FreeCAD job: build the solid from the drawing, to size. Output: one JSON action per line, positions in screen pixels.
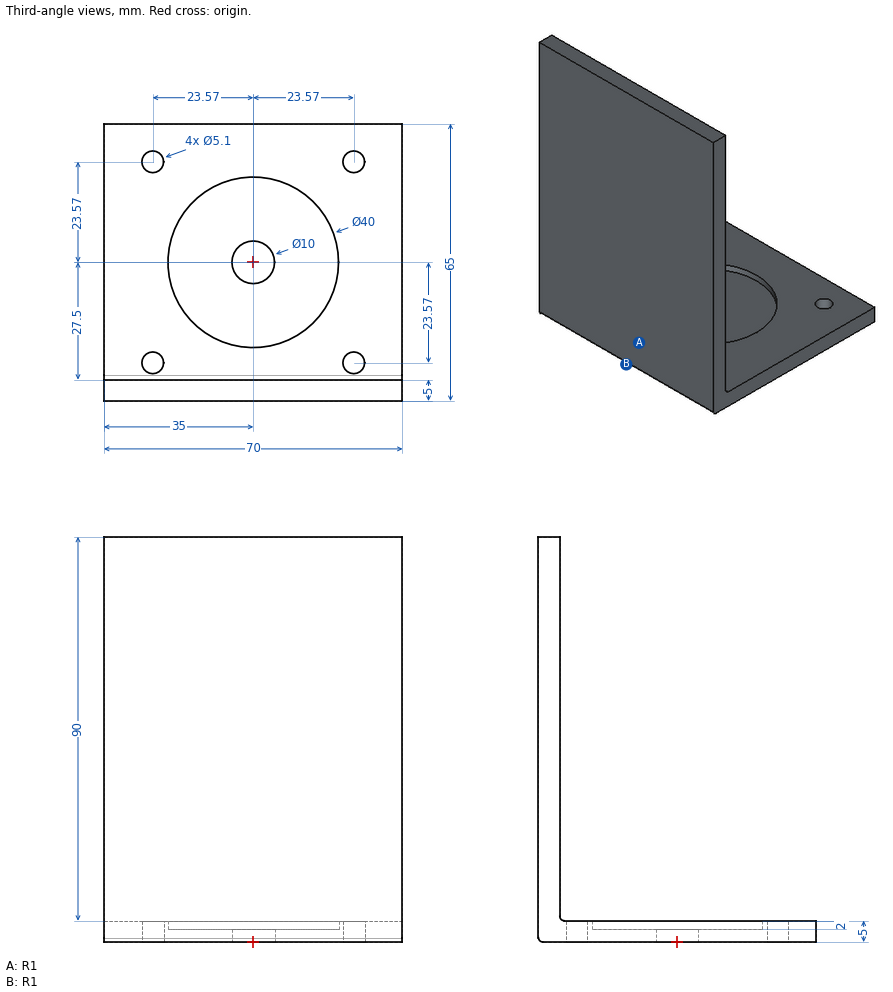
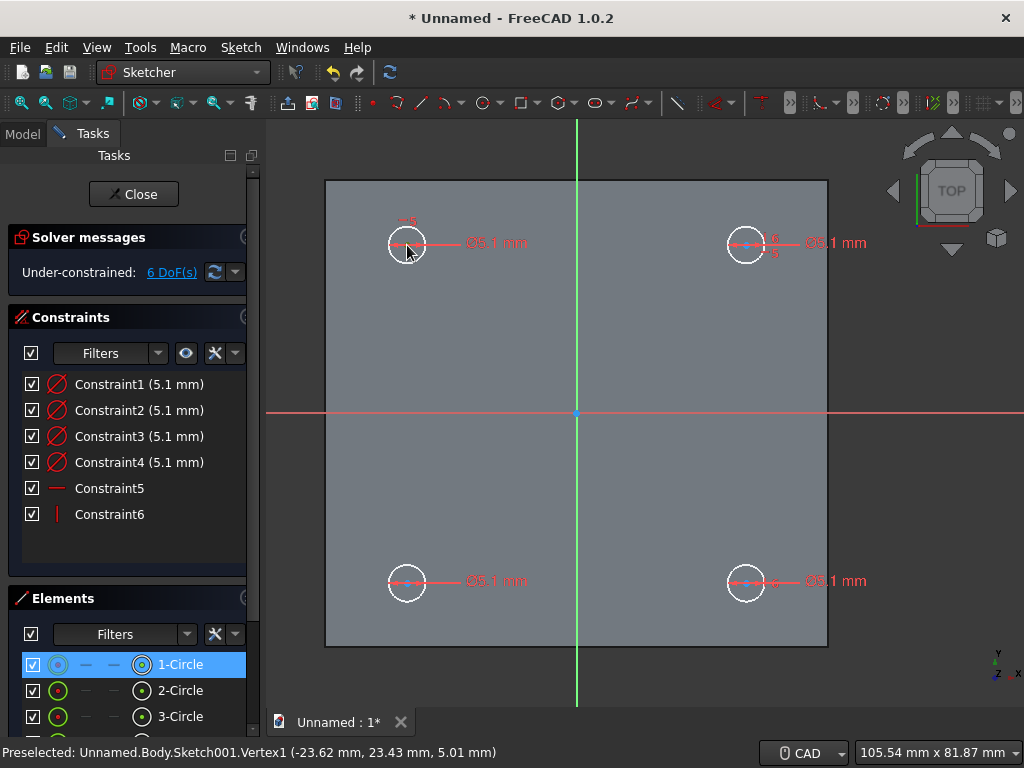
{"action": "left_click", "coordinate": [407, 583]}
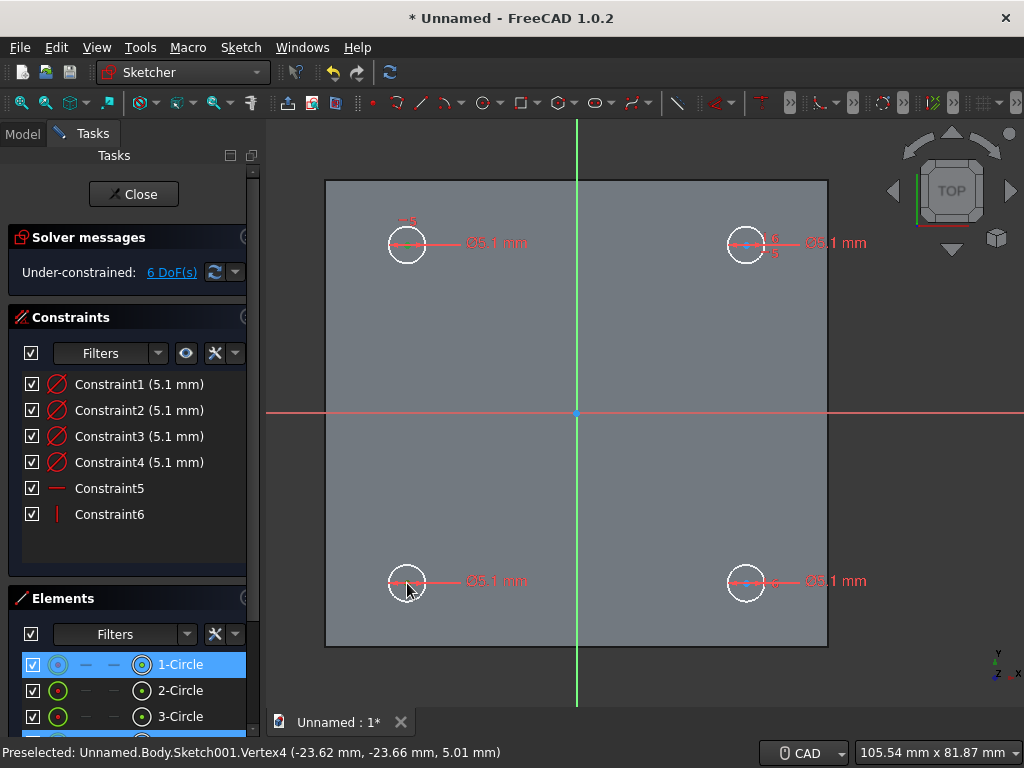
{"action": "key", "text": "v"}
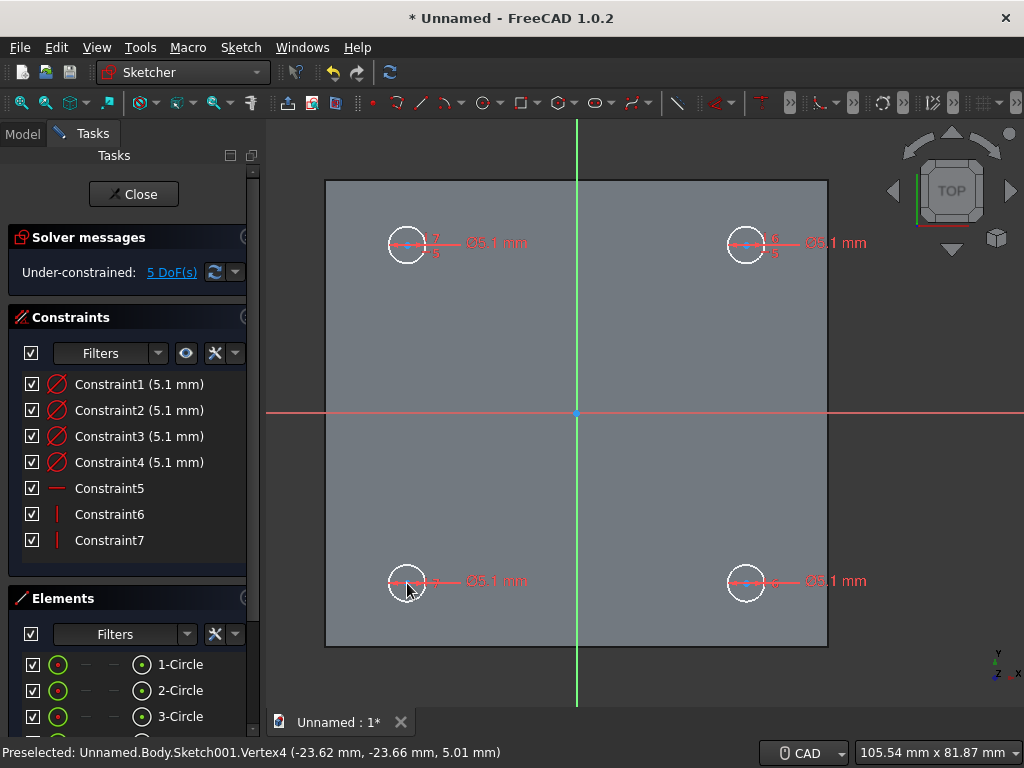
{"action": "left_click", "coordinate": [746, 583]}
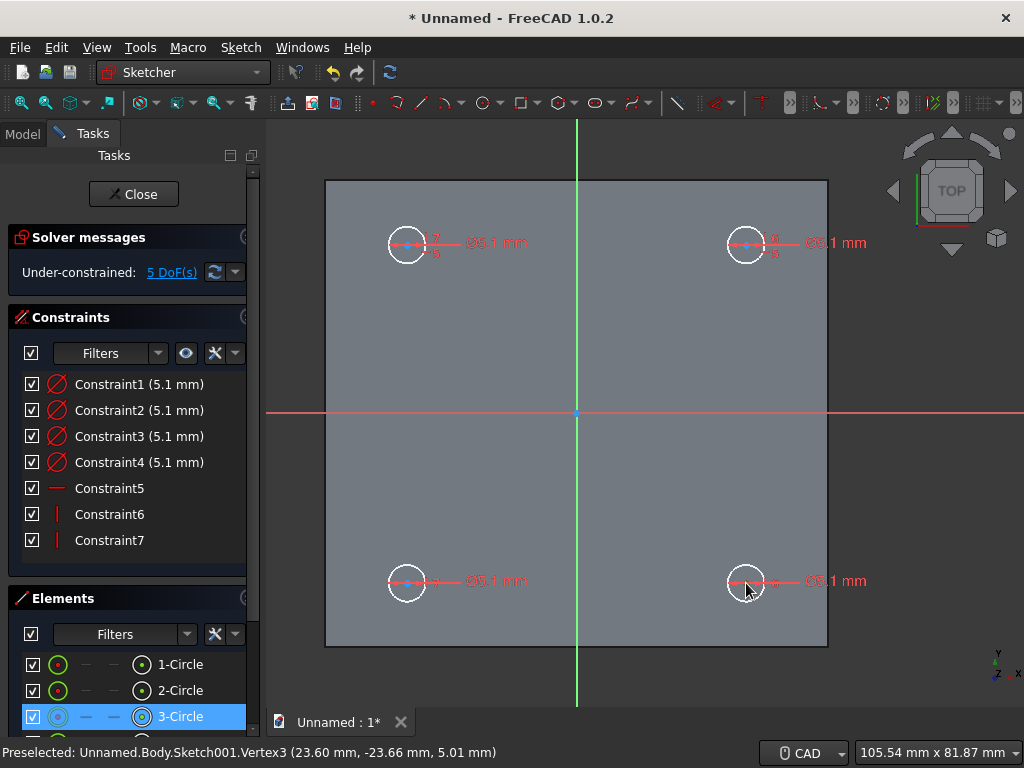
{"action": "left_click", "coordinate": [407, 583]}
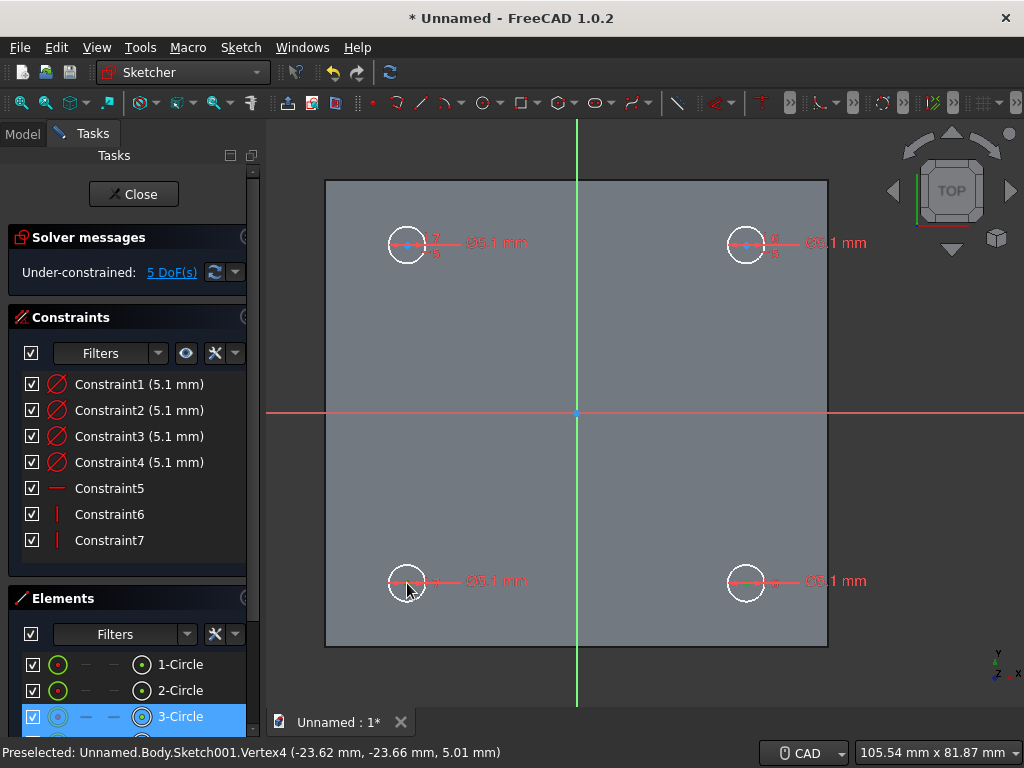
{"action": "key", "text": "h"}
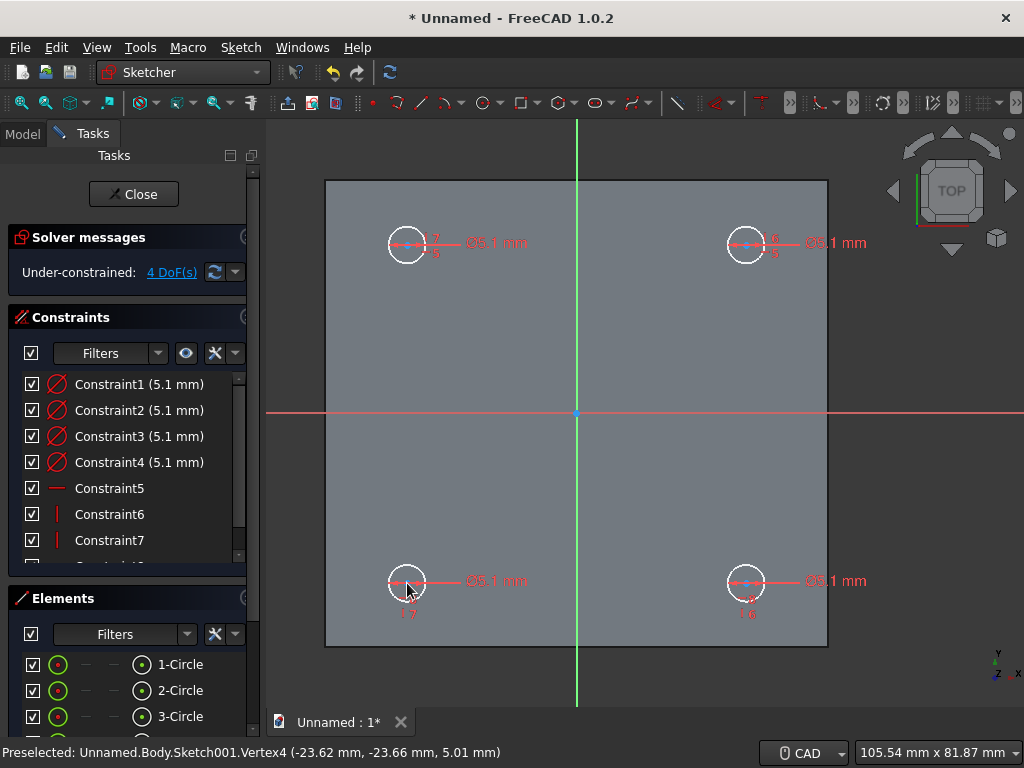
{"action": "left_click", "coordinate": [716, 104]}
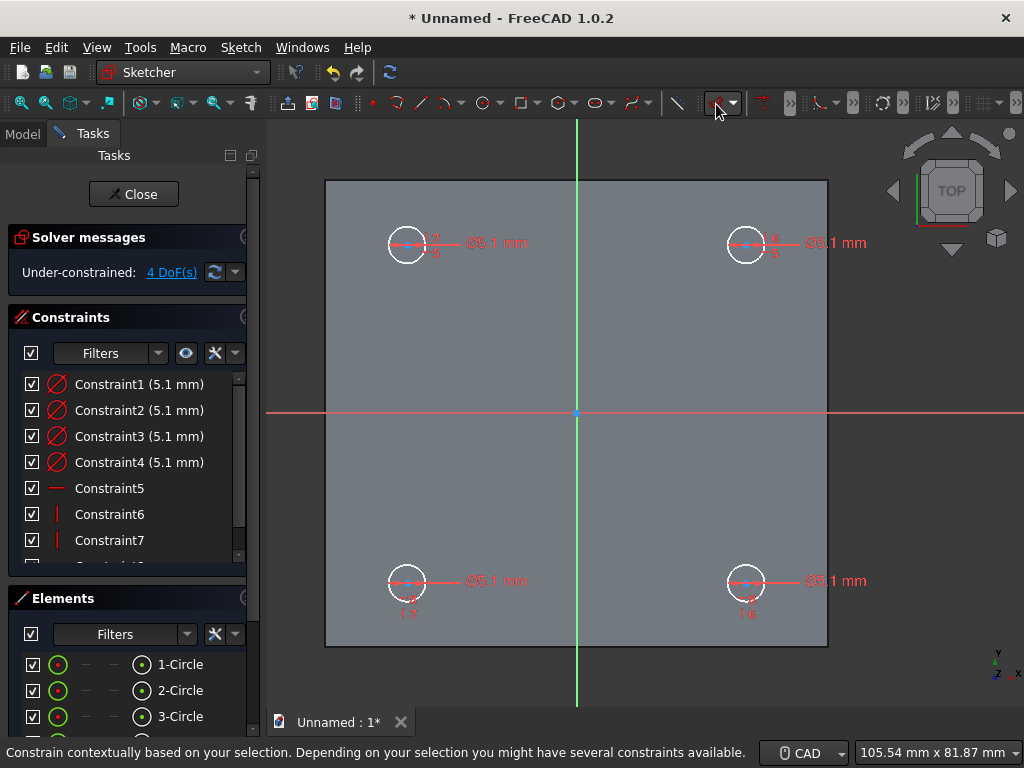
{"action": "left_click", "coordinate": [407, 245]}
{"action": "left_click", "coordinate": [492, 211]}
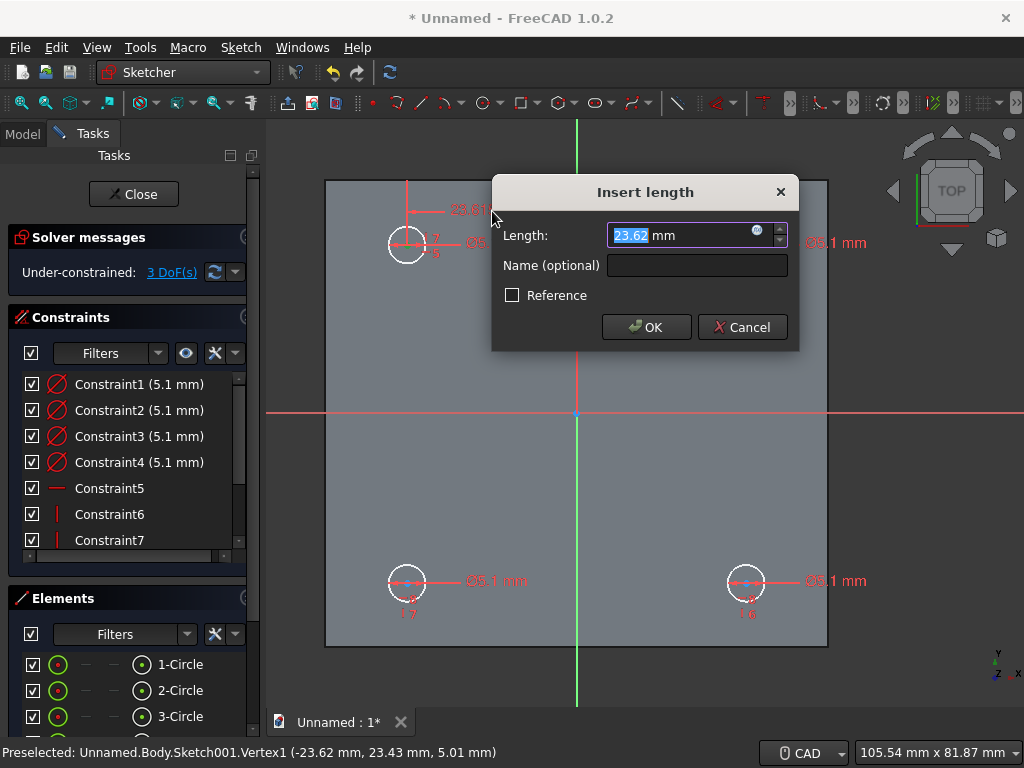
{"action": "type", "text": "23.57"}
{"action": "key", "text": "Return"}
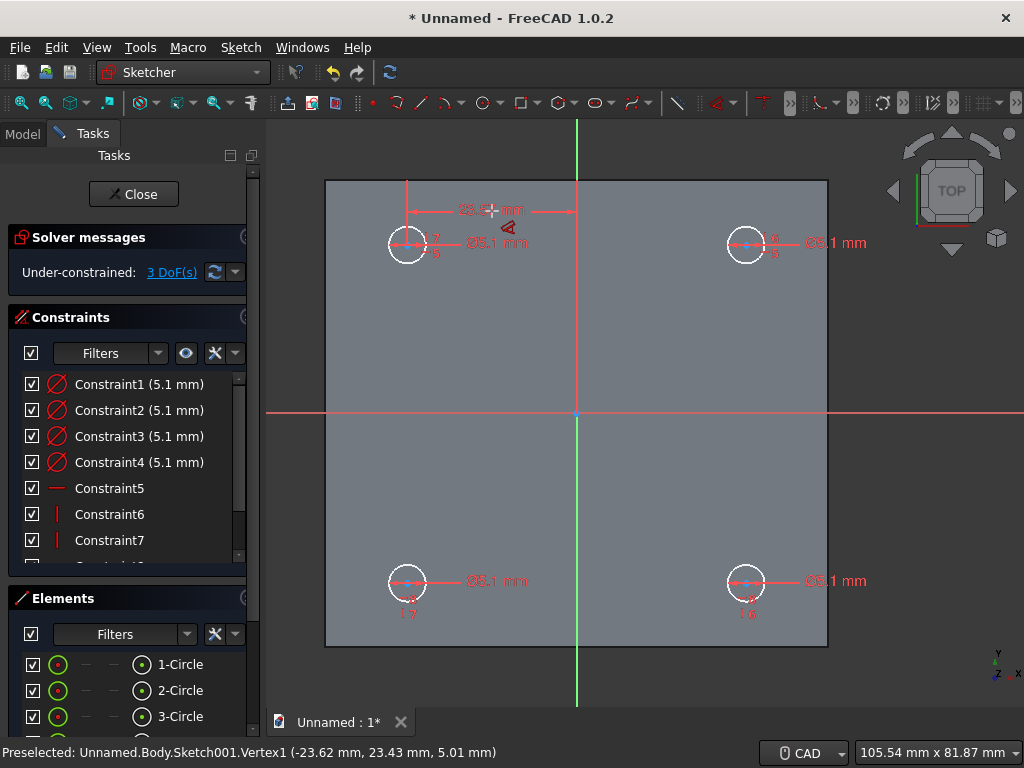
{"action": "left_click", "coordinate": [407, 245]}
{"action": "left_click", "coordinate": [373, 329]}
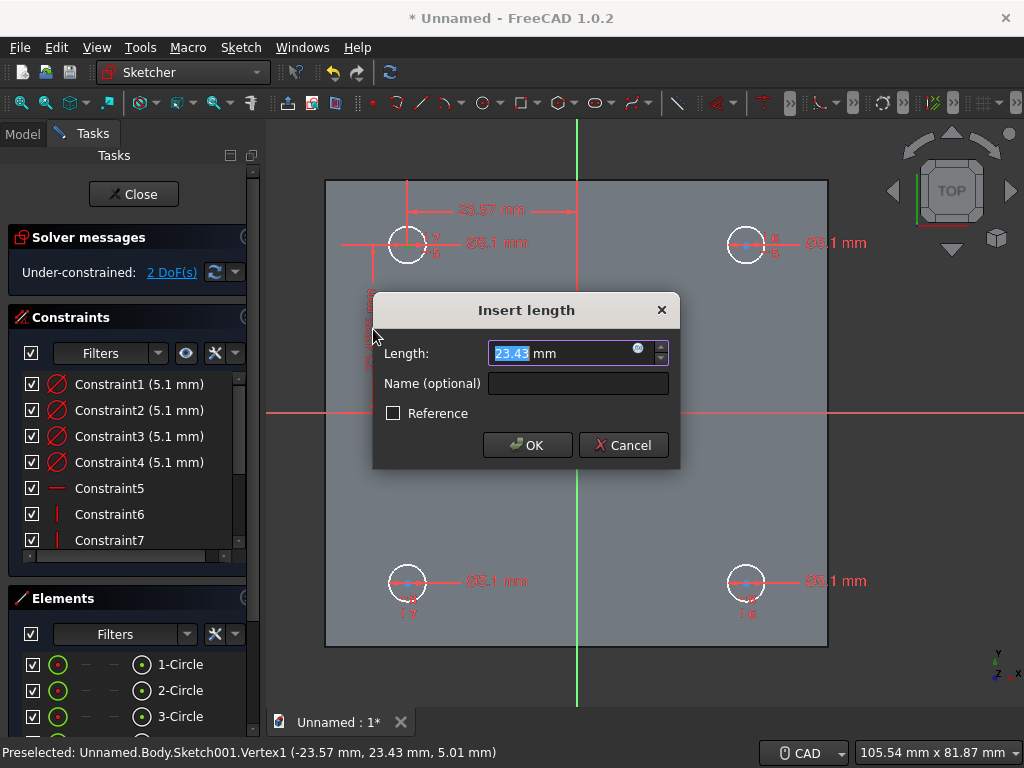
{"action": "type", "text": "23.57"}
{"action": "key", "text": "Return"}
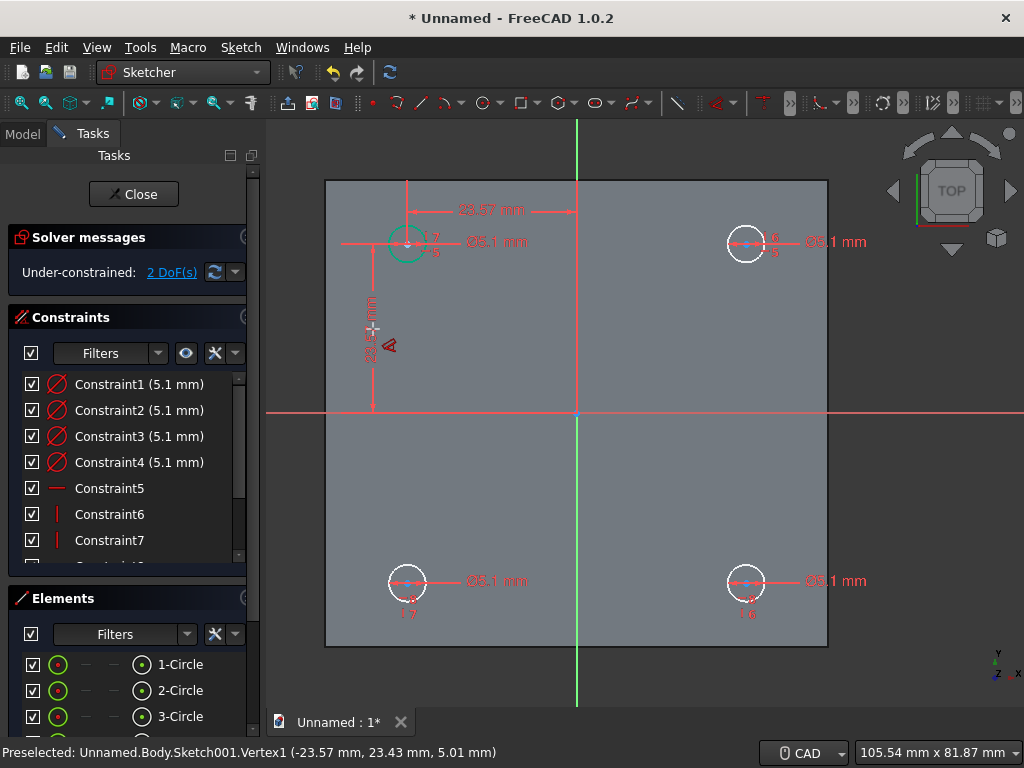
{"action": "left_click", "coordinate": [746, 244]}
{"action": "left_click", "coordinate": [661, 210]}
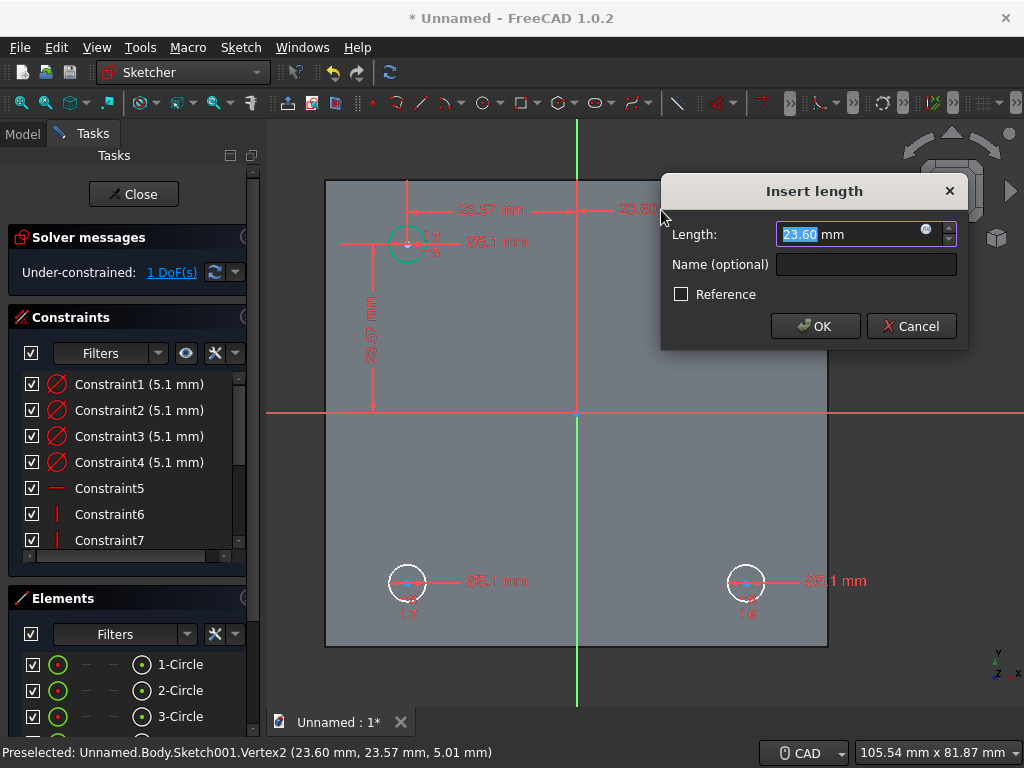
{"action": "type", "text": "23.57"}
{"action": "key", "text": "Return"}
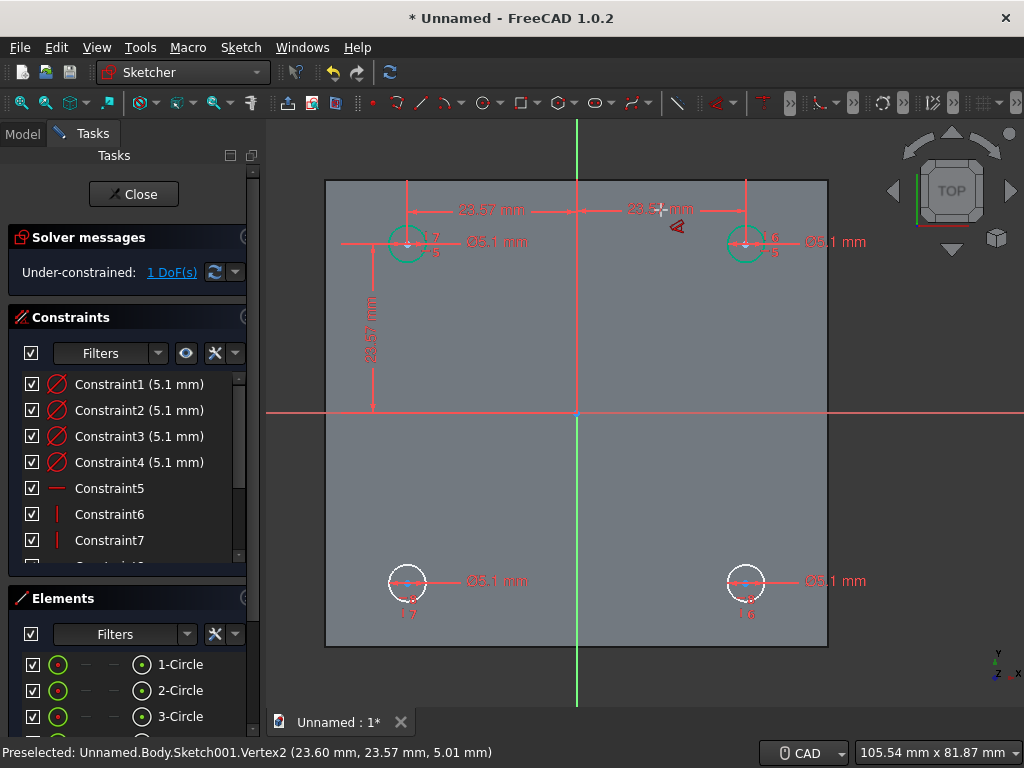
{"action": "left_click", "coordinate": [746, 583]}
{"action": "left_click", "coordinate": [780, 498]}